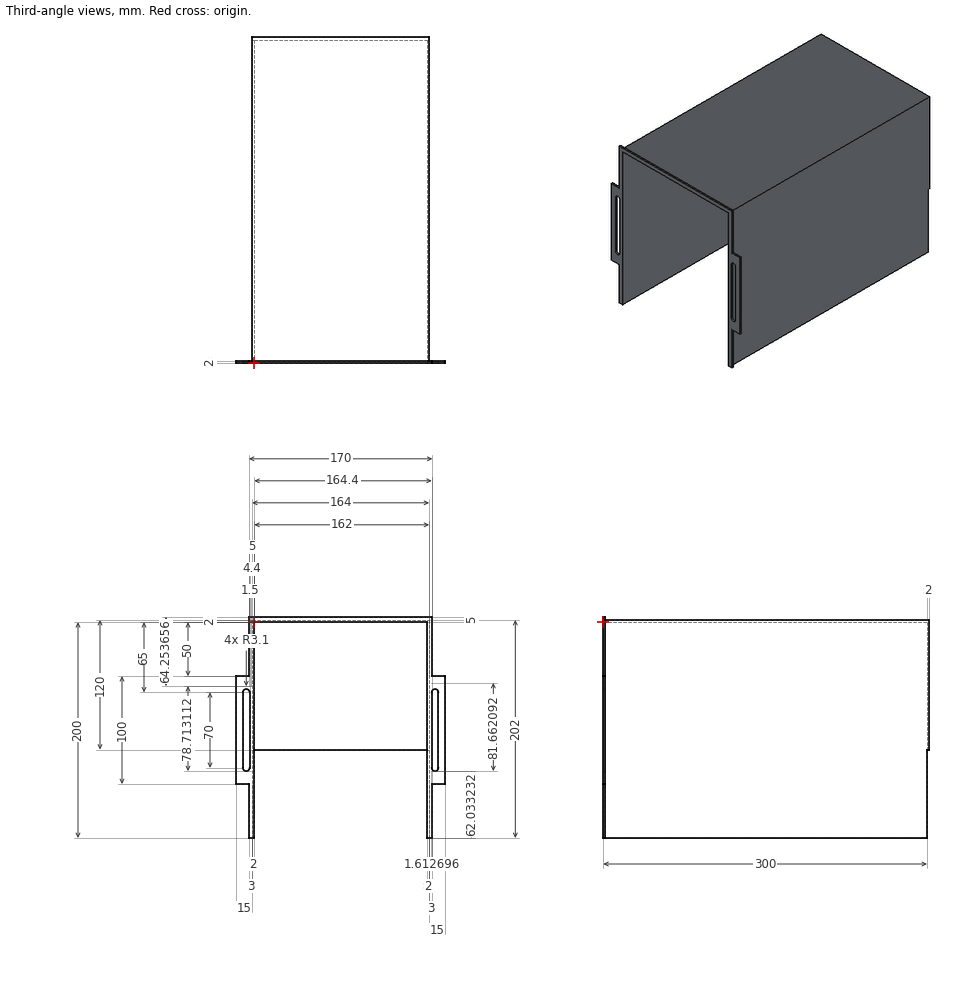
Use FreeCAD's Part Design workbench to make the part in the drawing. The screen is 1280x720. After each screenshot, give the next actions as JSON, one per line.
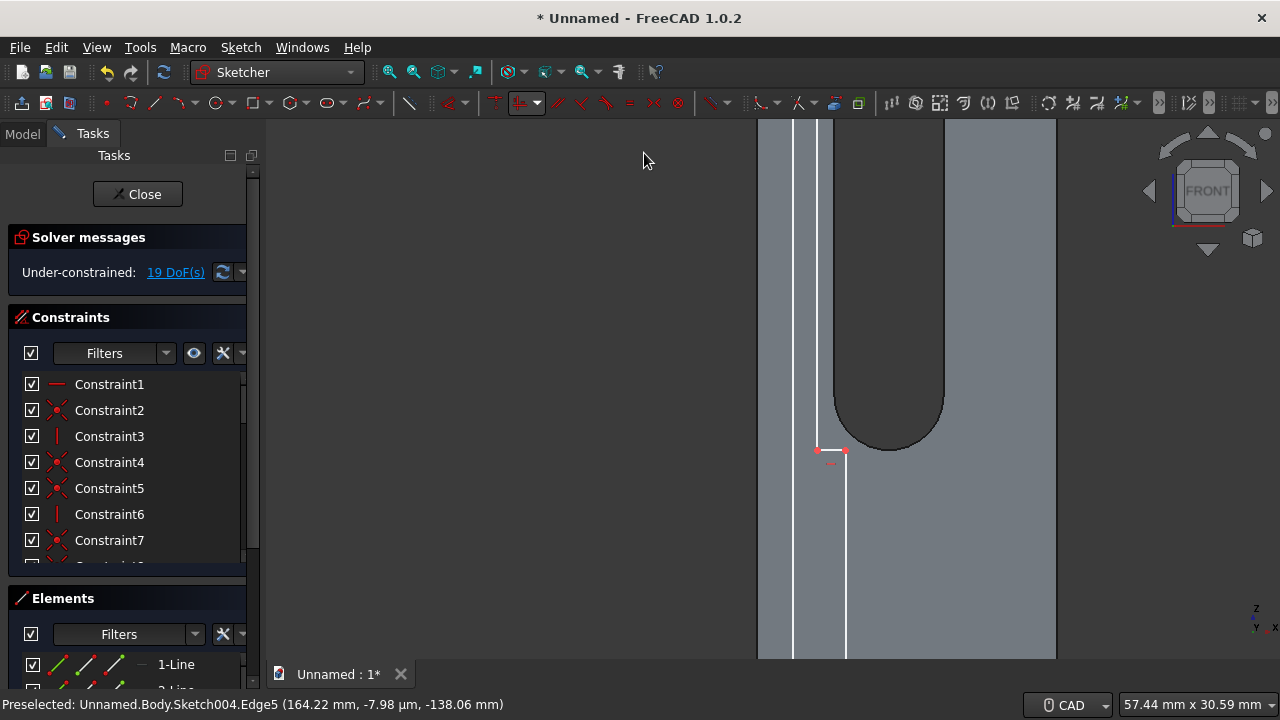
{"action": "scroll", "coordinate": [840, 454], "scroll_direction": "down", "scroll_amount": 12}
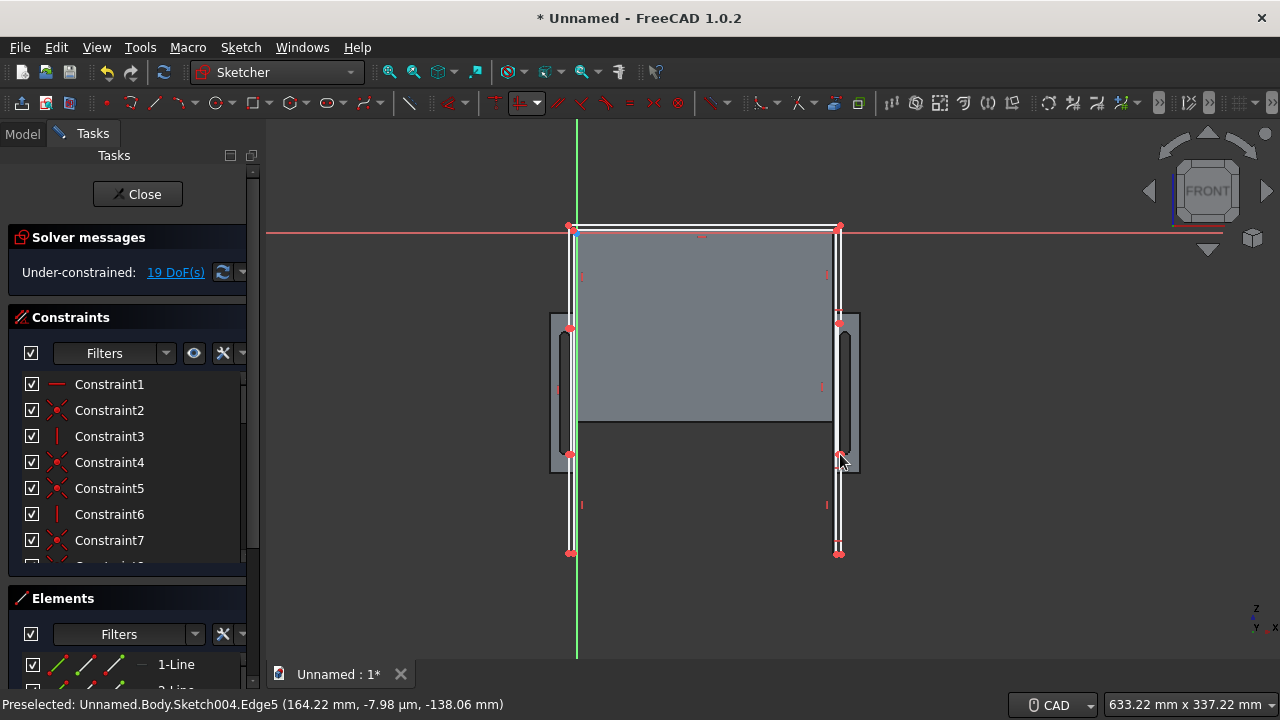
{"action": "scroll", "coordinate": [570, 328], "scroll_direction": "up", "scroll_amount": 14}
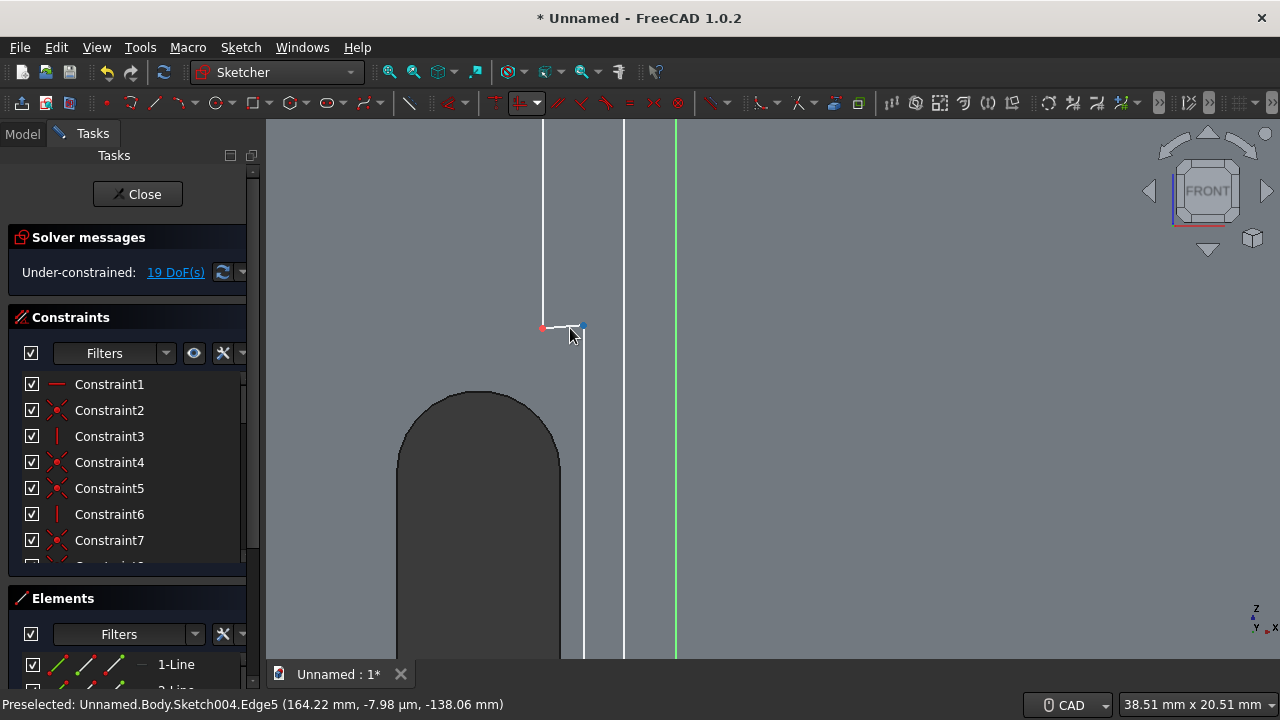
{"action": "left_click", "coordinate": [559, 327]}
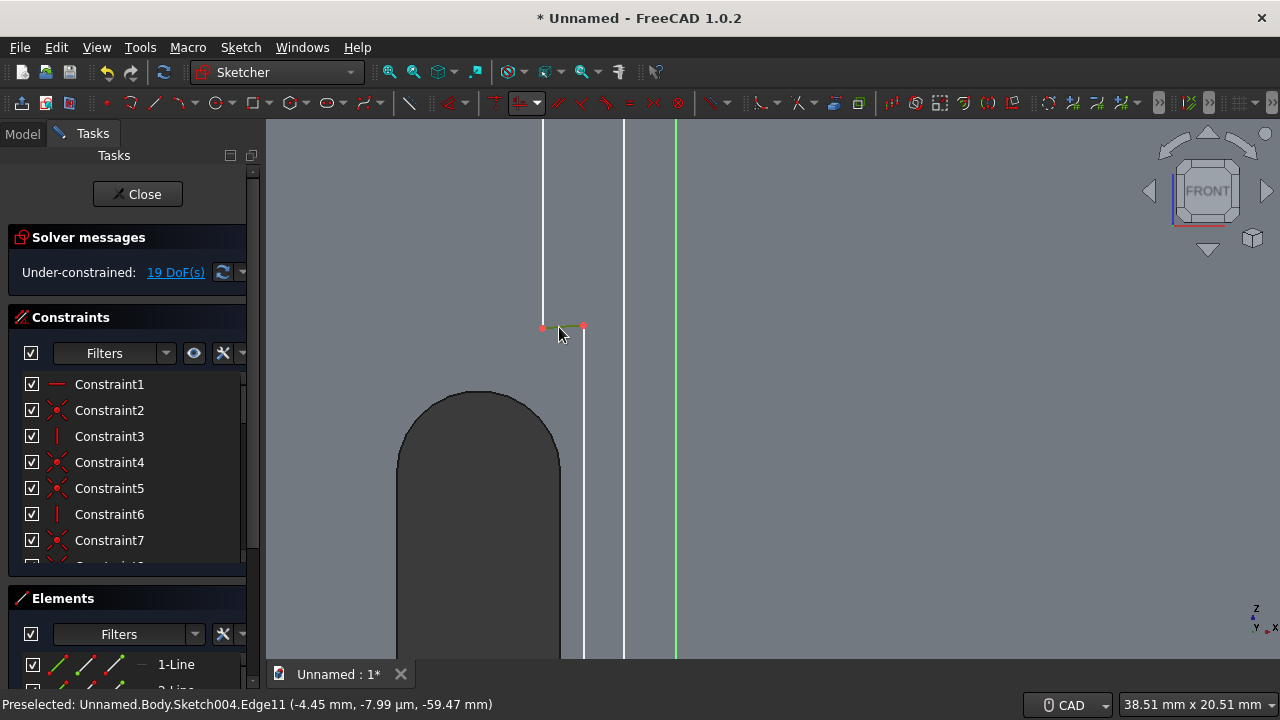
{"action": "left_click", "coordinate": [540, 104]}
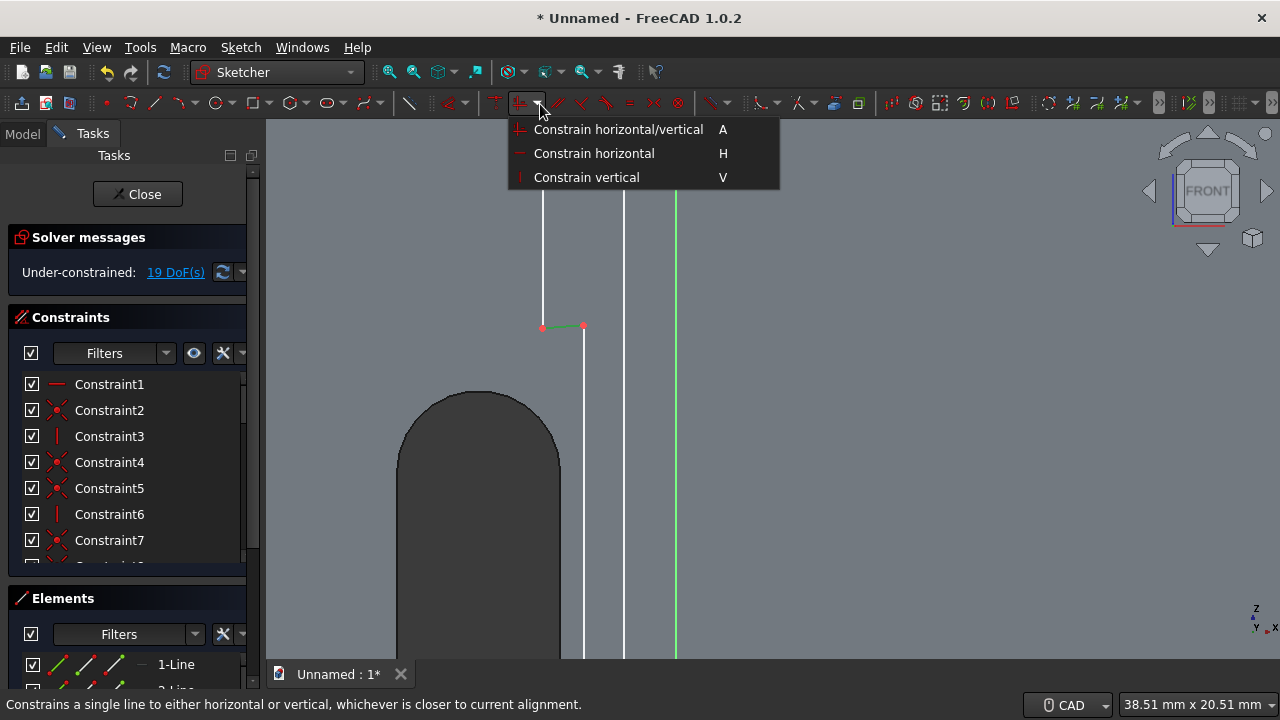
{"action": "left_click", "coordinate": [644, 153]}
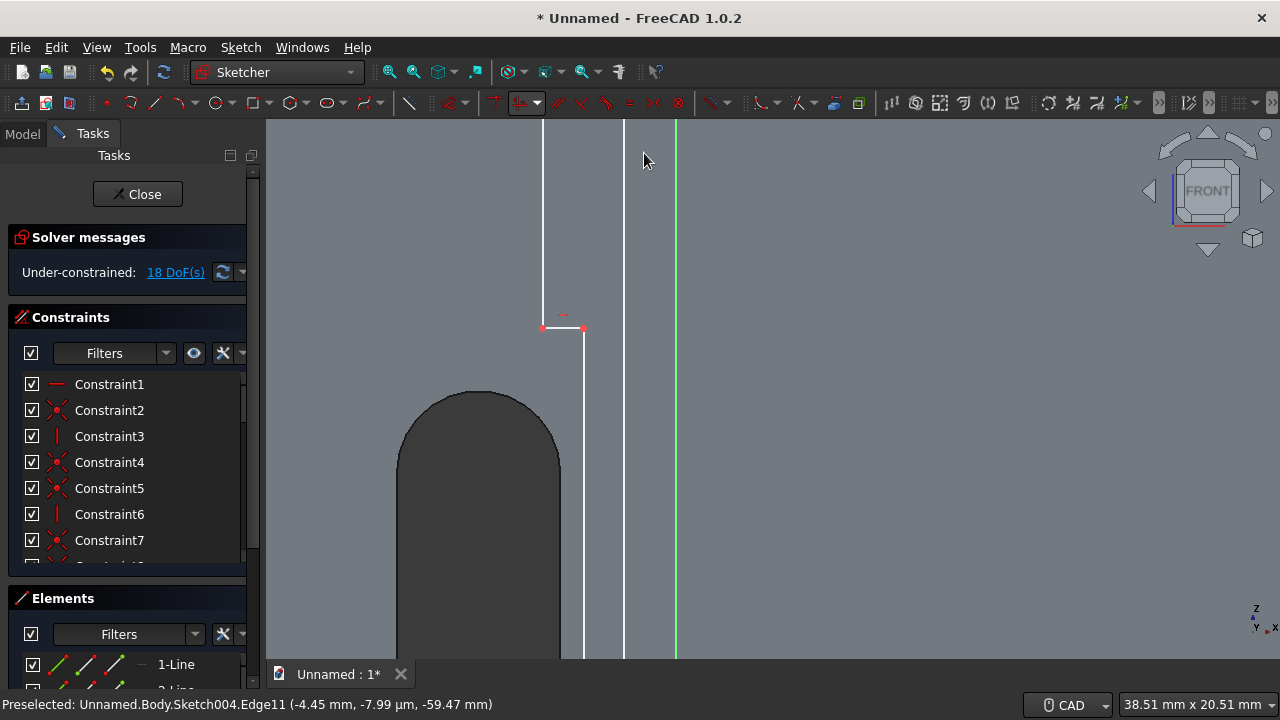
{"action": "scroll", "coordinate": [570, 328], "scroll_direction": "down", "scroll_amount": 14}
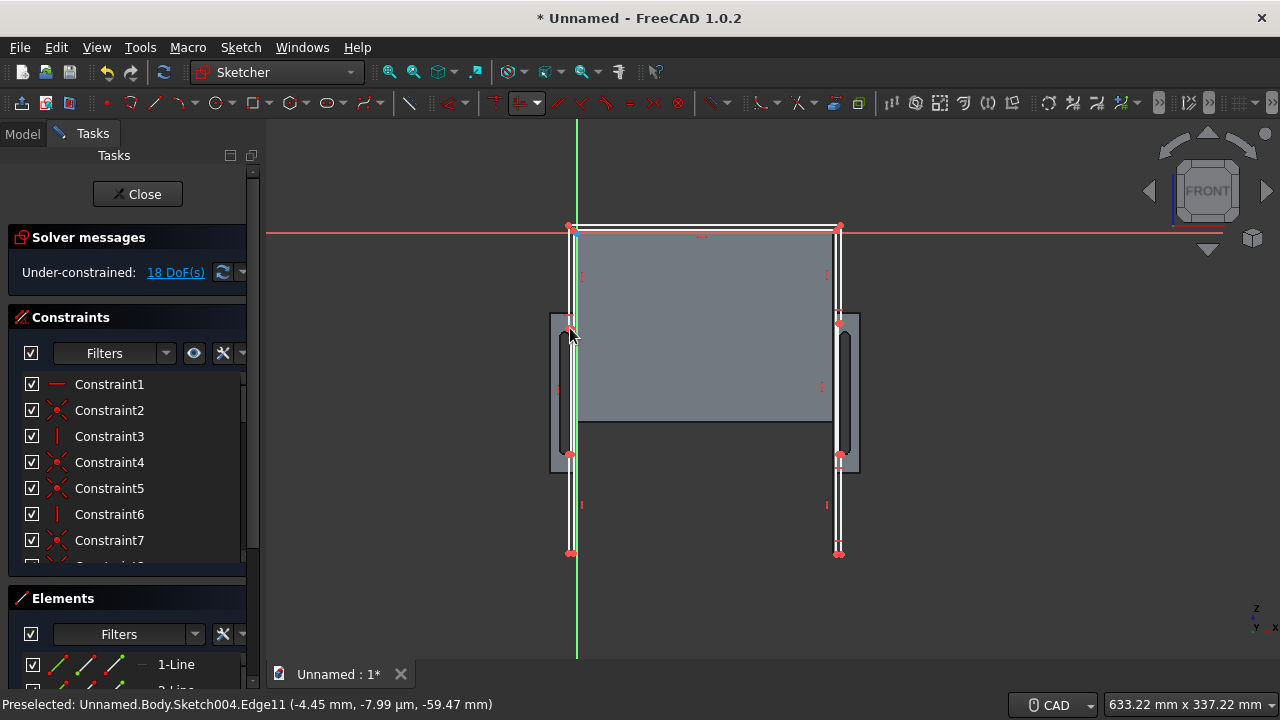
{"action": "scroll", "coordinate": [570, 454], "scroll_direction": "up", "scroll_amount": 14}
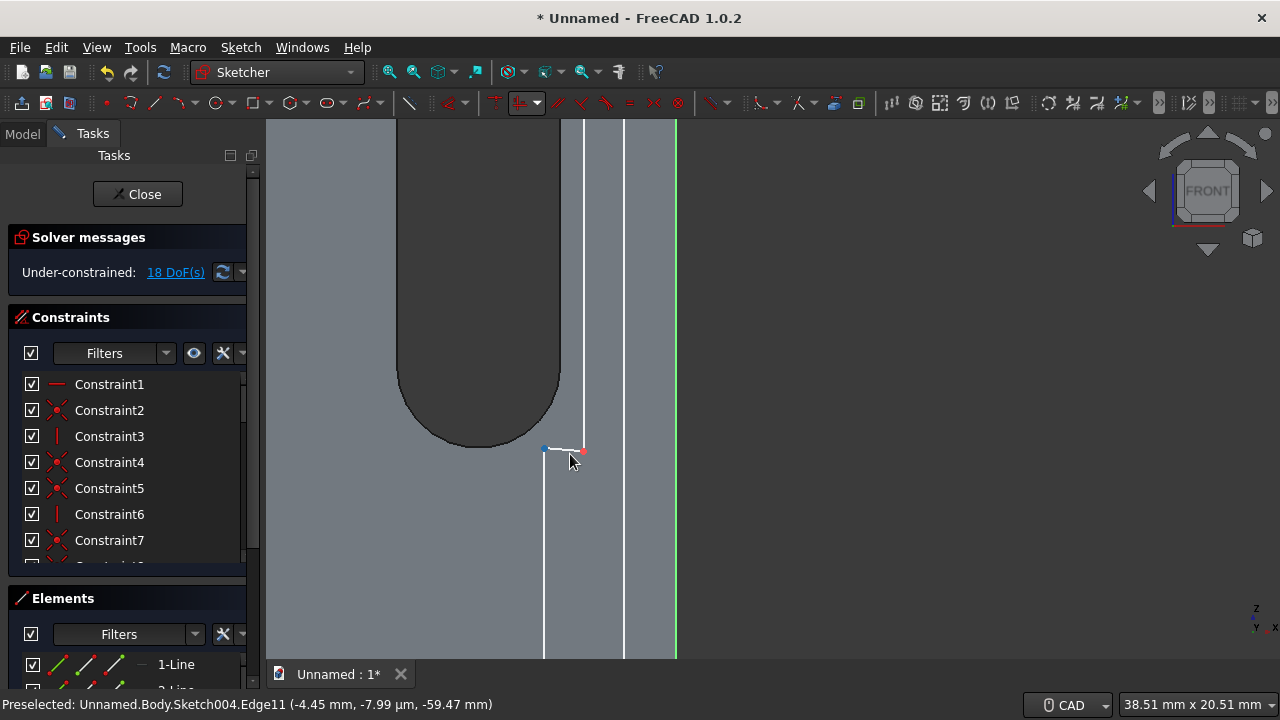
{"action": "left_click", "coordinate": [572, 450]}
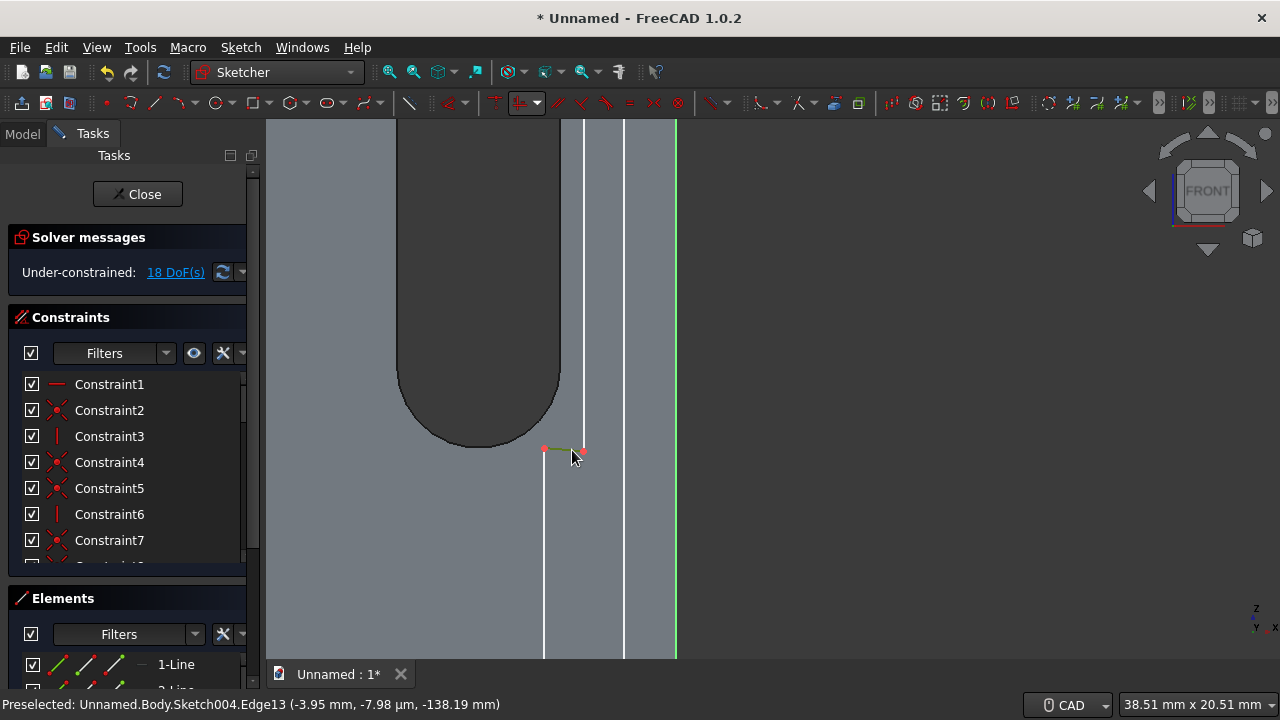
{"action": "left_click", "coordinate": [540, 104]}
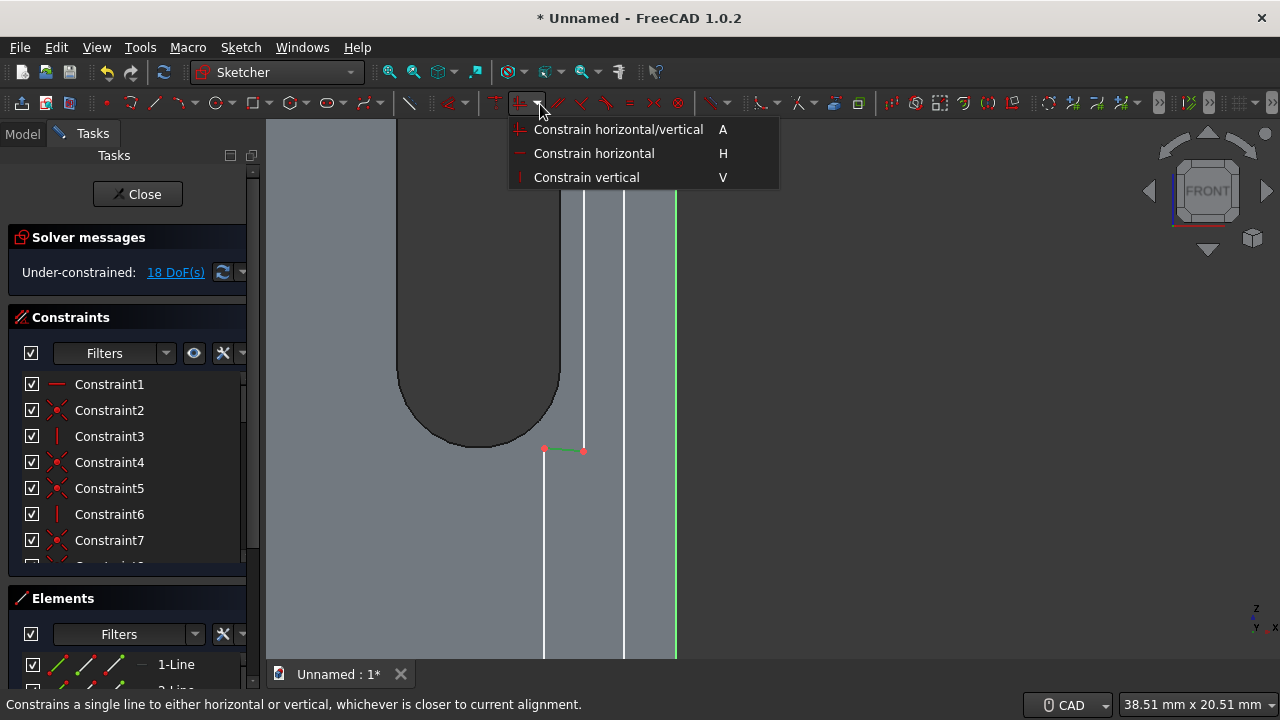
{"action": "left_click", "coordinate": [644, 153]}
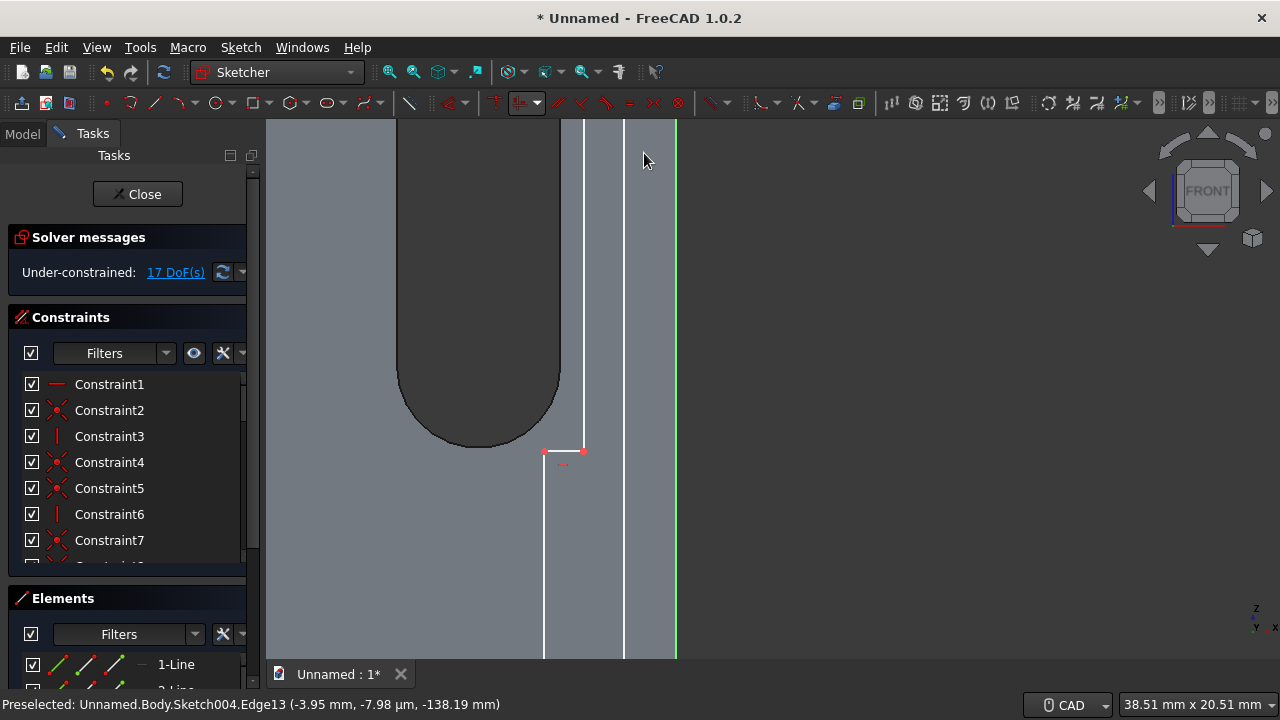
{"action": "scroll", "coordinate": [570, 454], "scroll_direction": "down", "scroll_amount": 14}